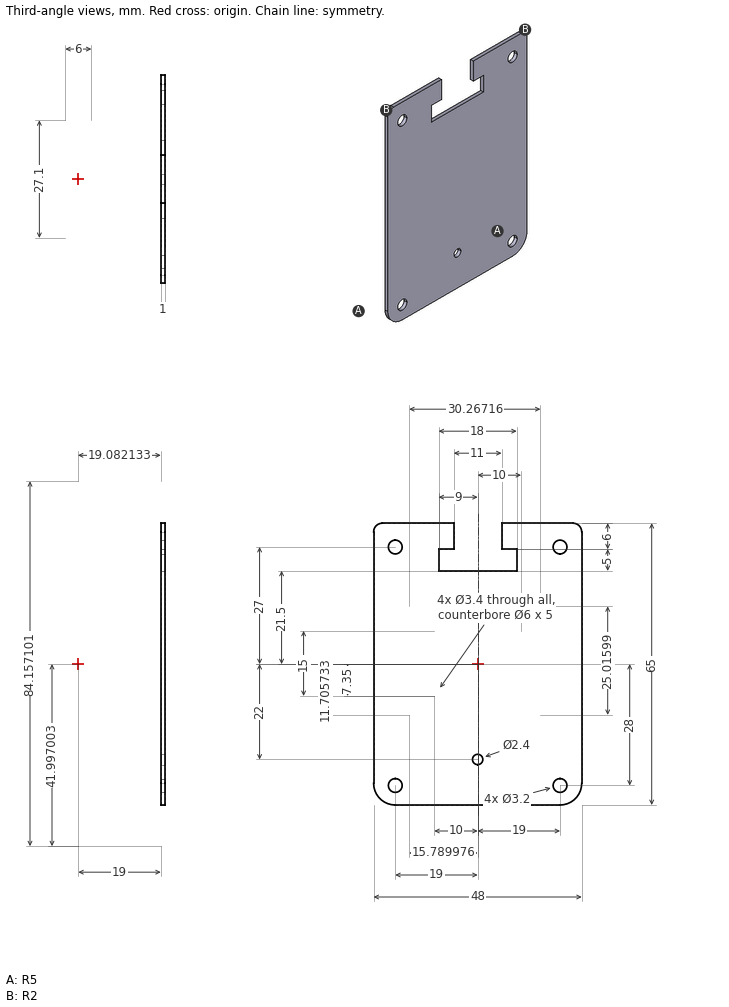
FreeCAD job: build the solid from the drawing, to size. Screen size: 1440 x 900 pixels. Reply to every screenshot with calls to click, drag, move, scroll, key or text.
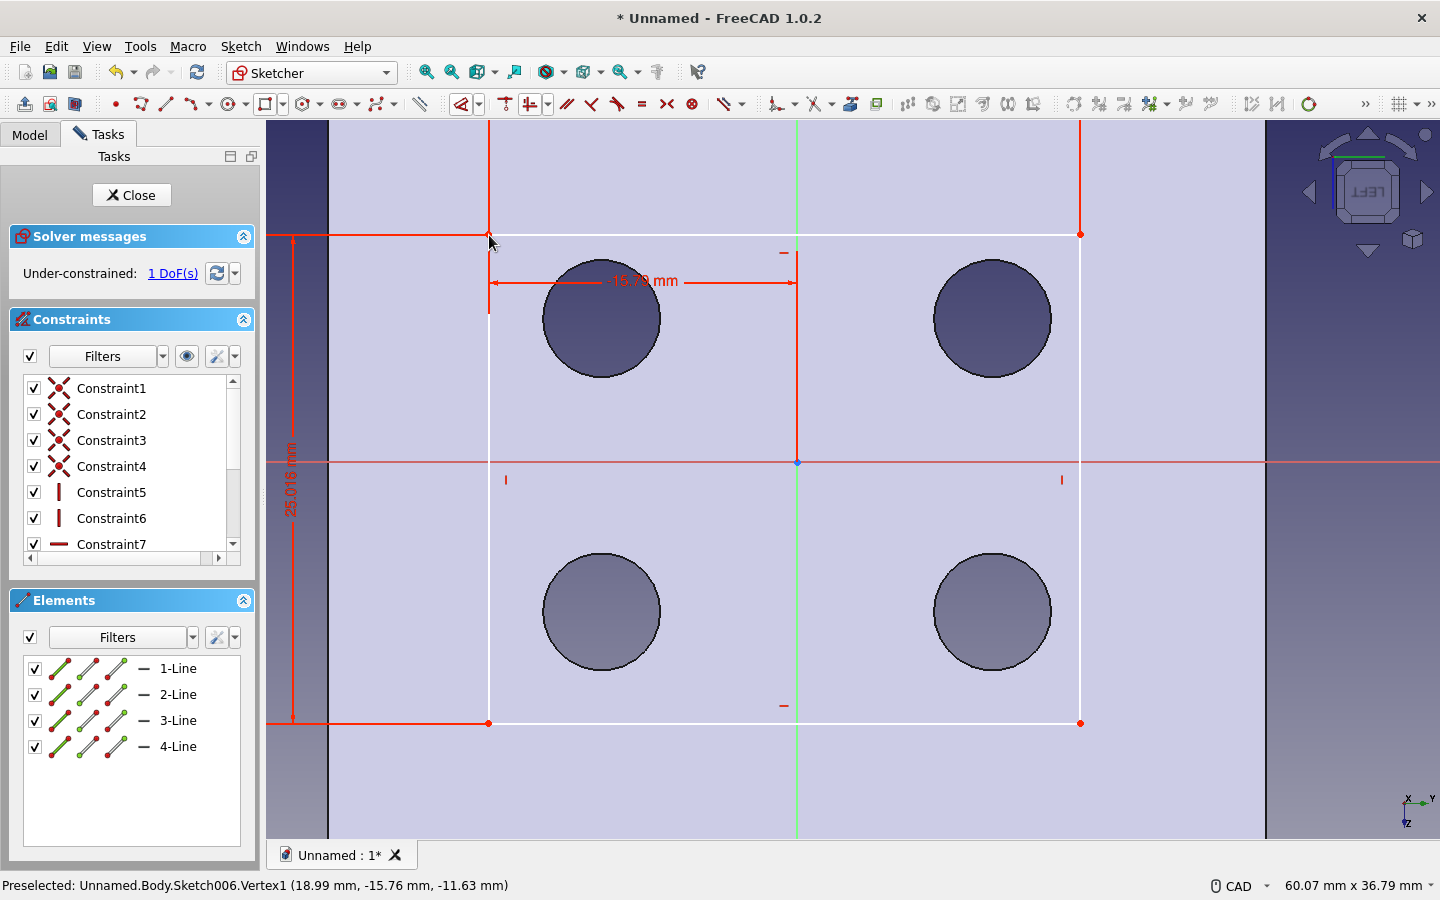
click(489, 235)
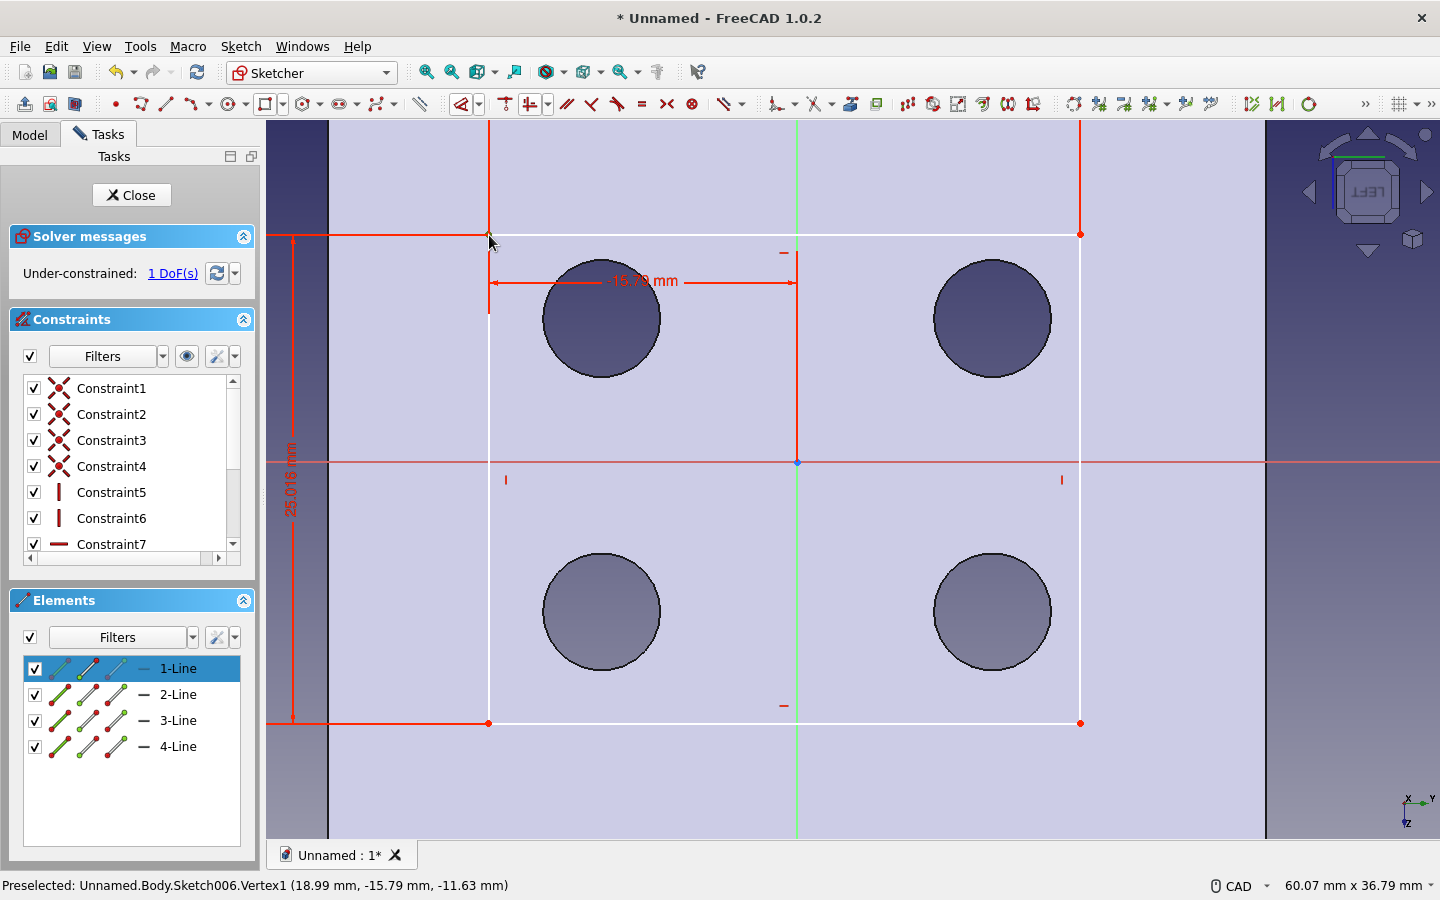
key(i)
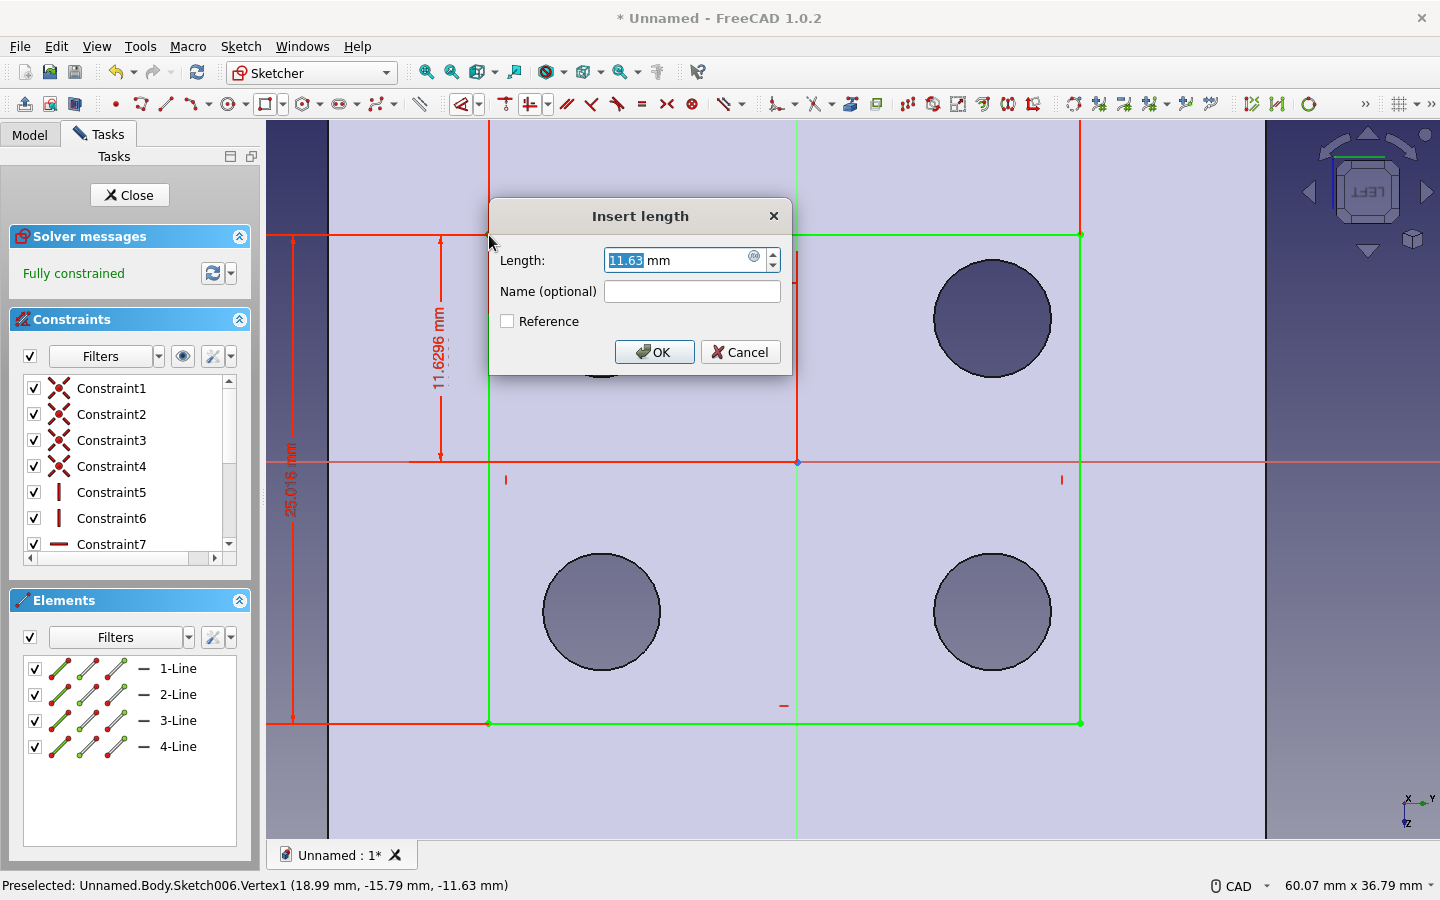
text(11.705733)
key(Return)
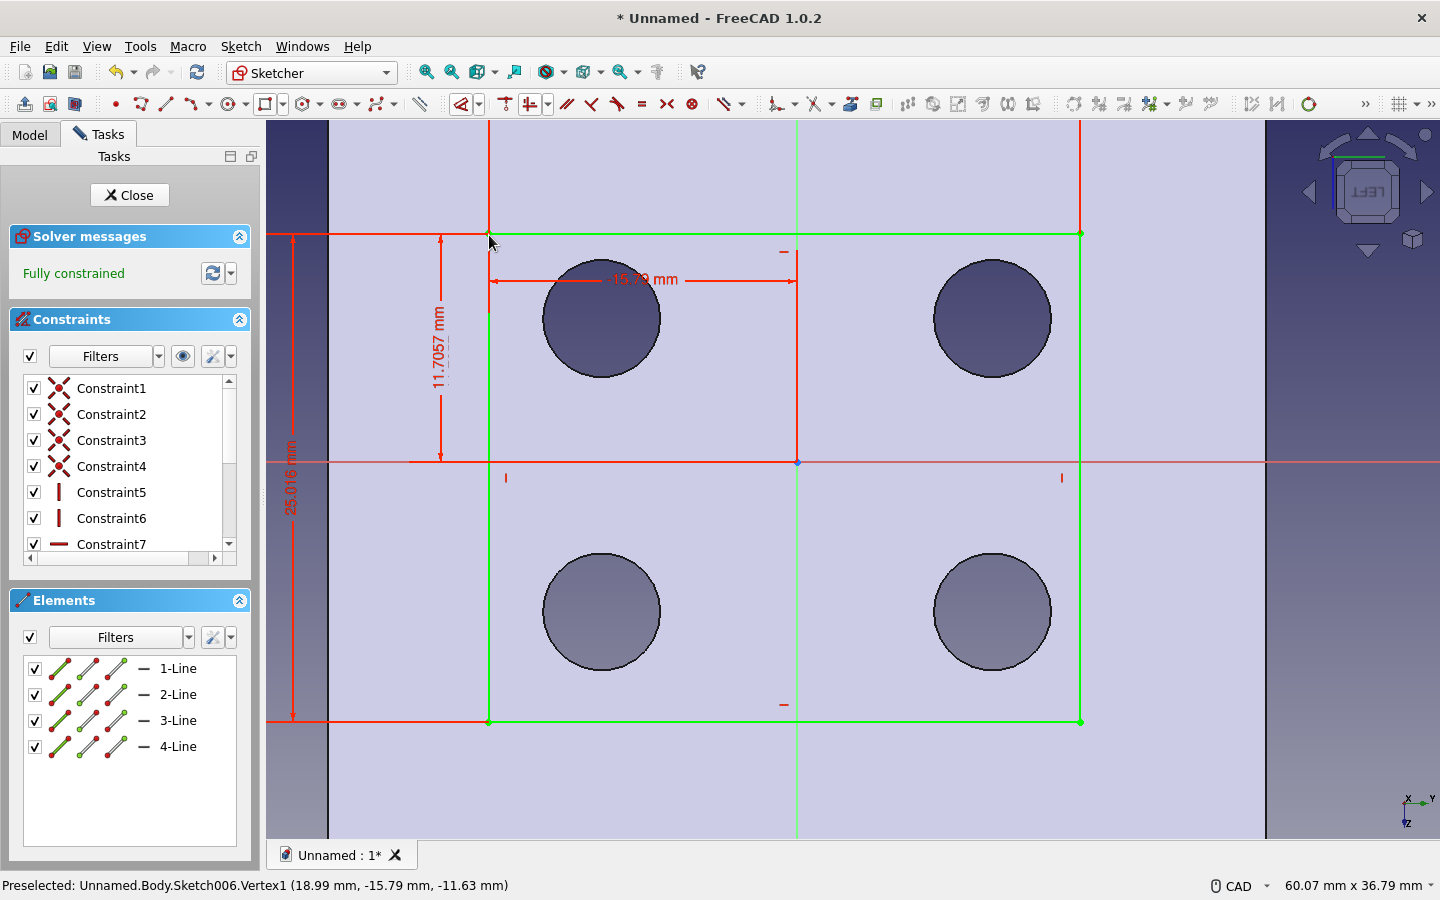
click(130, 195)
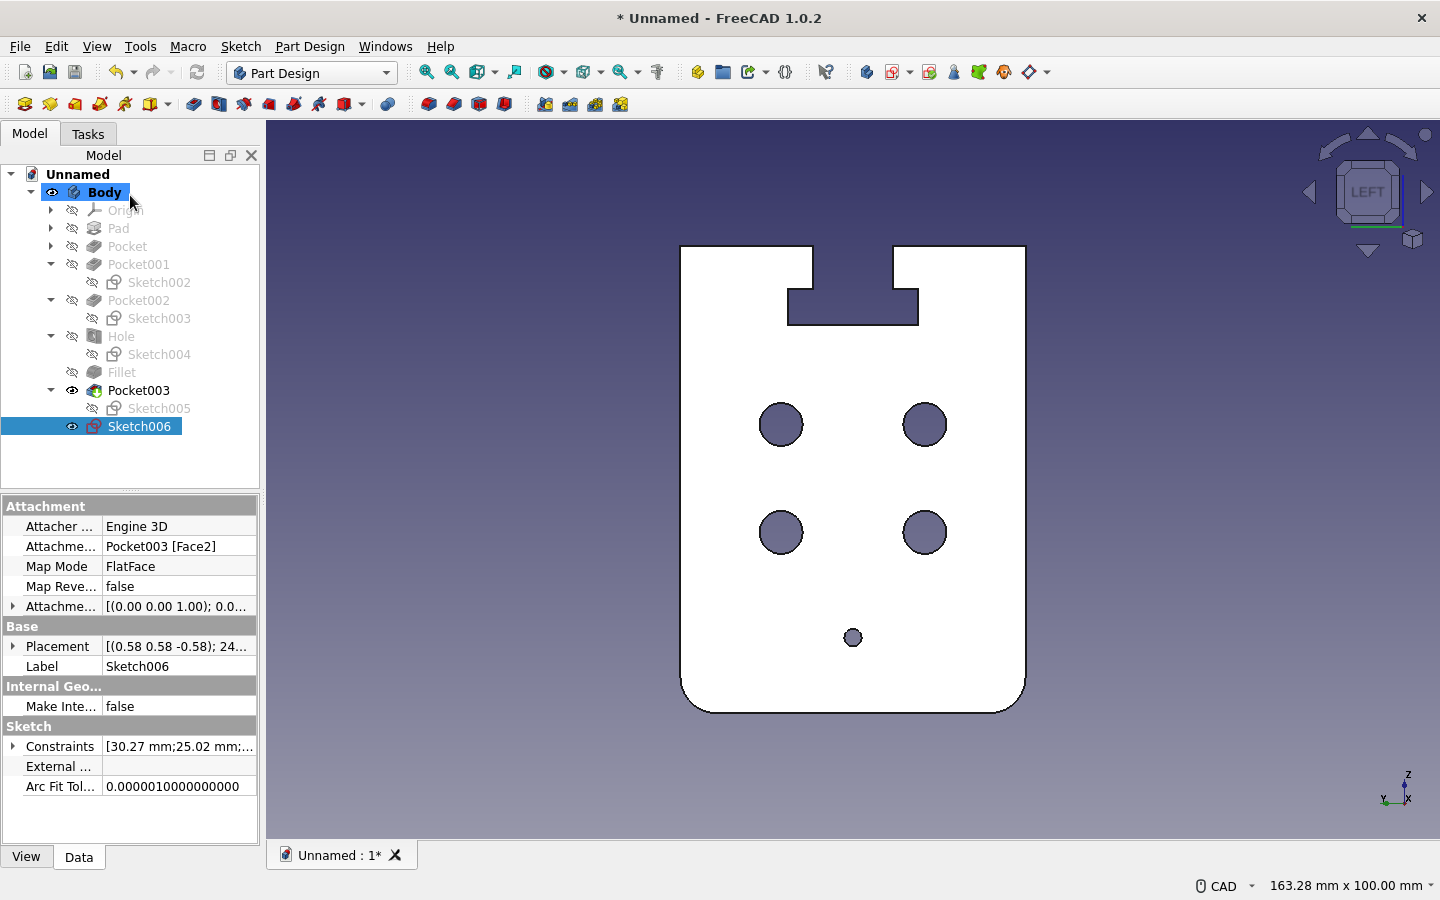
click(25, 104)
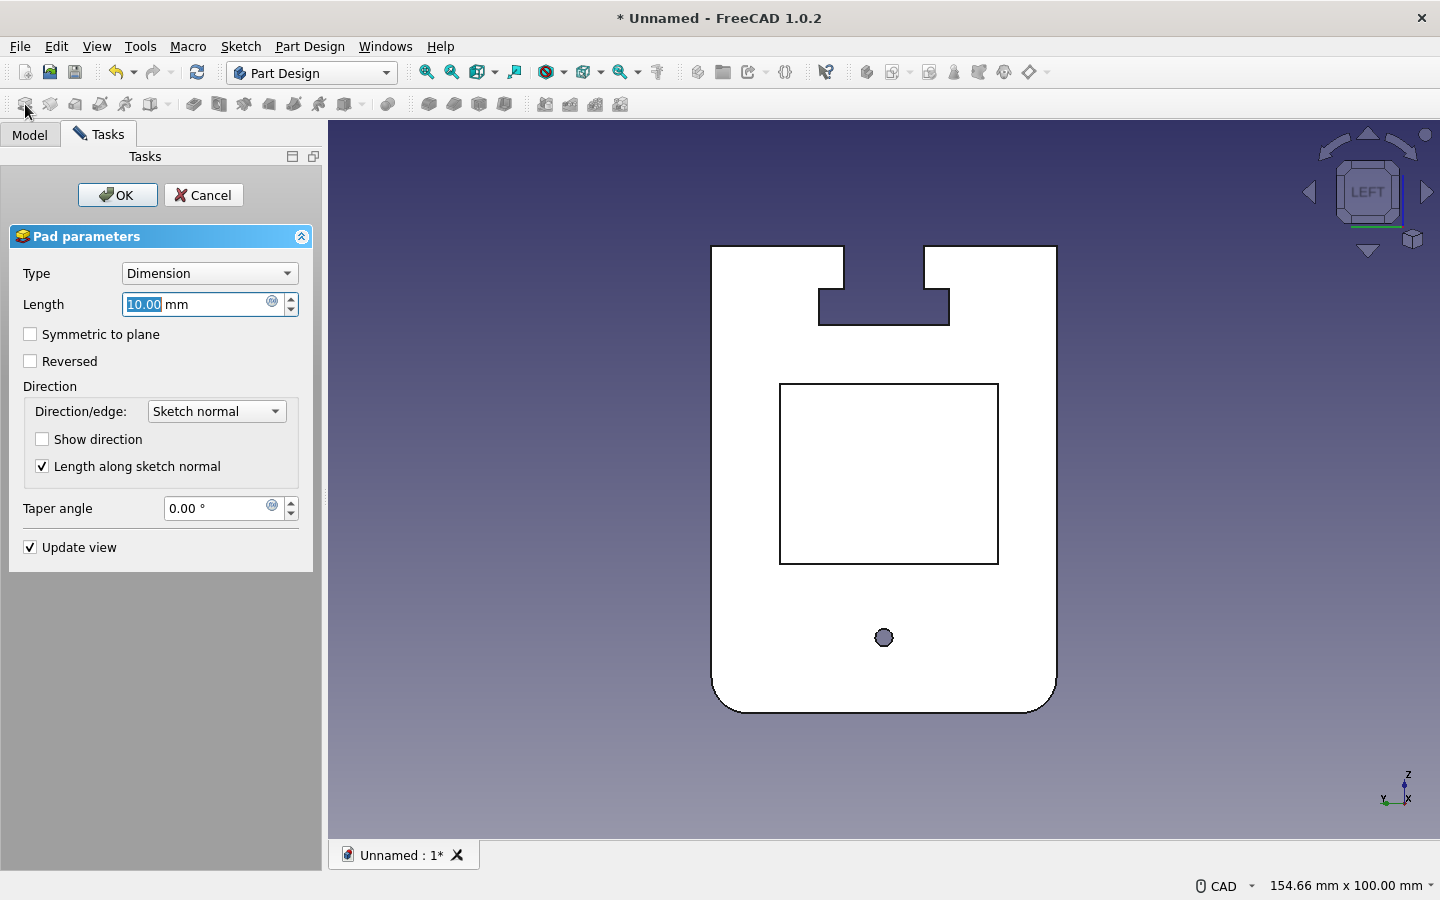
text(1)
key(Tab)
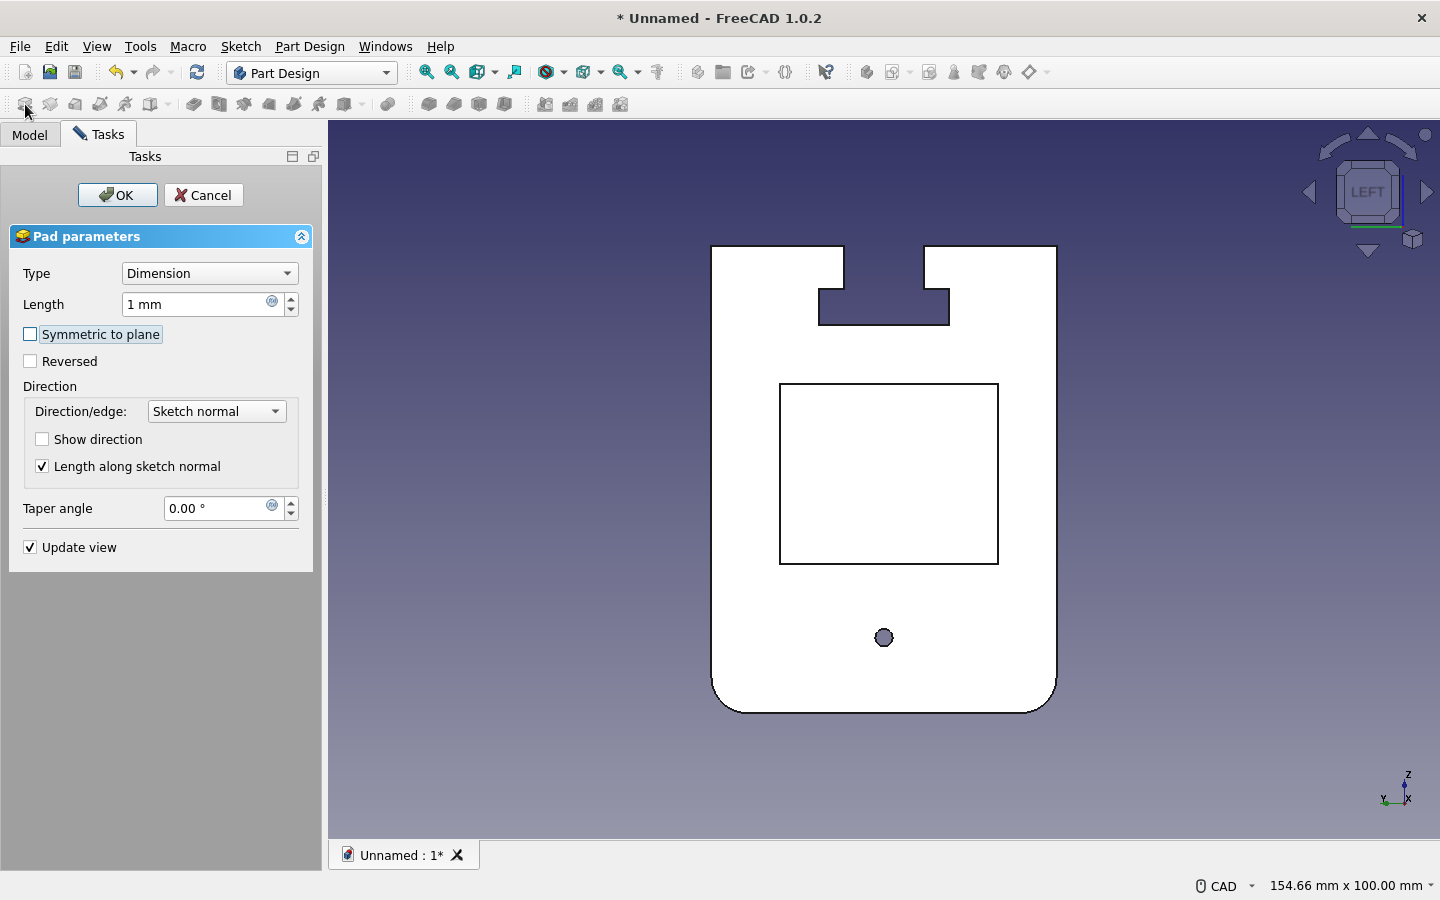
click(31, 361)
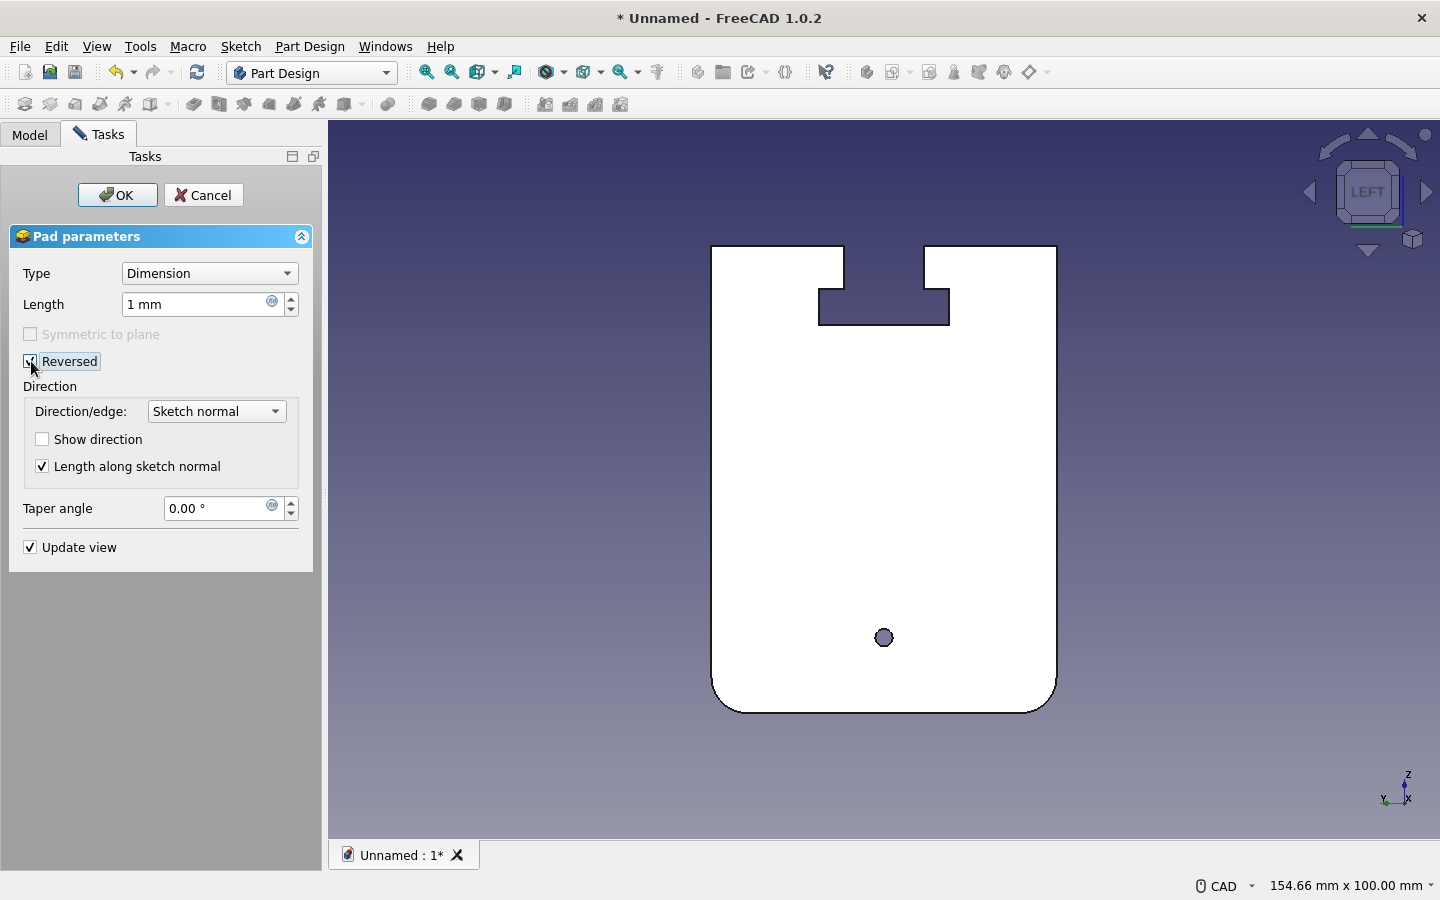
click(118, 195)